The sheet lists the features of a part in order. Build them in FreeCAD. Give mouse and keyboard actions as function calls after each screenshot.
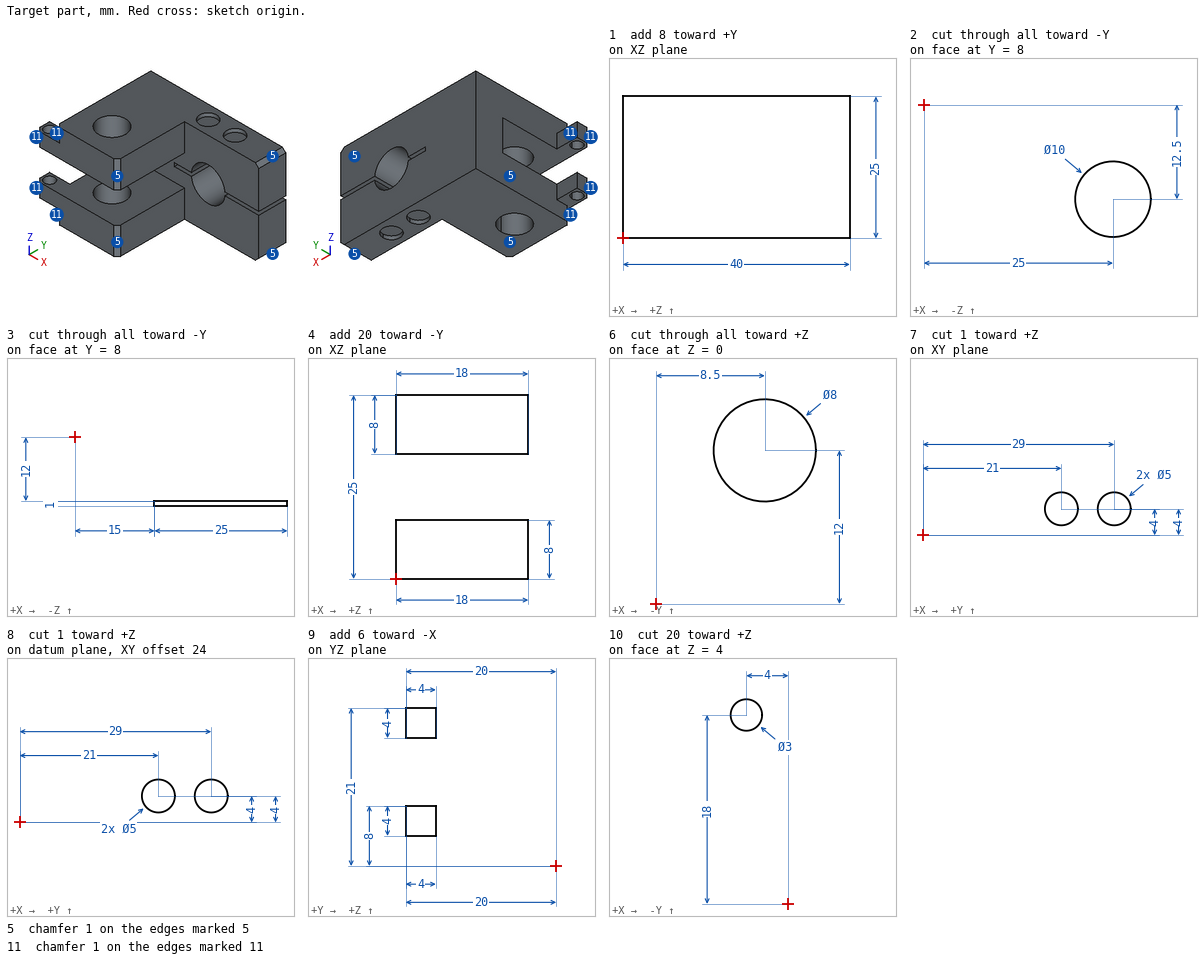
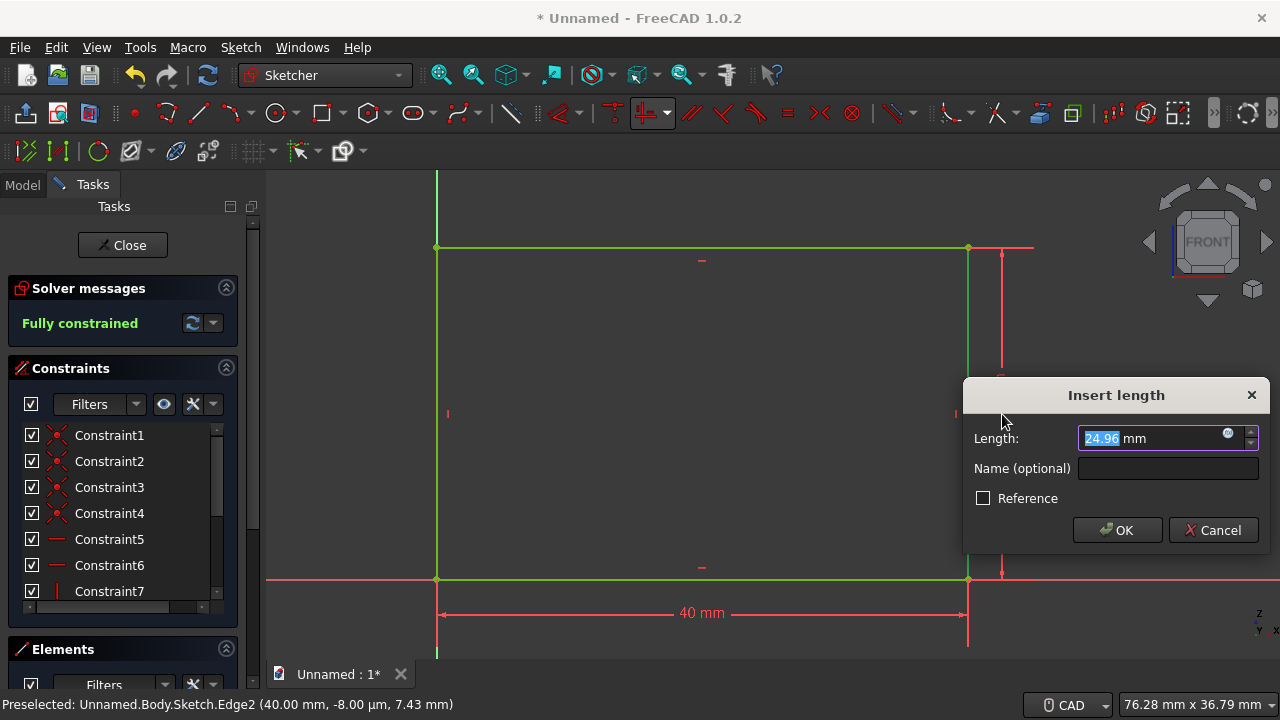
text(25)
key(Return)
key(Escape)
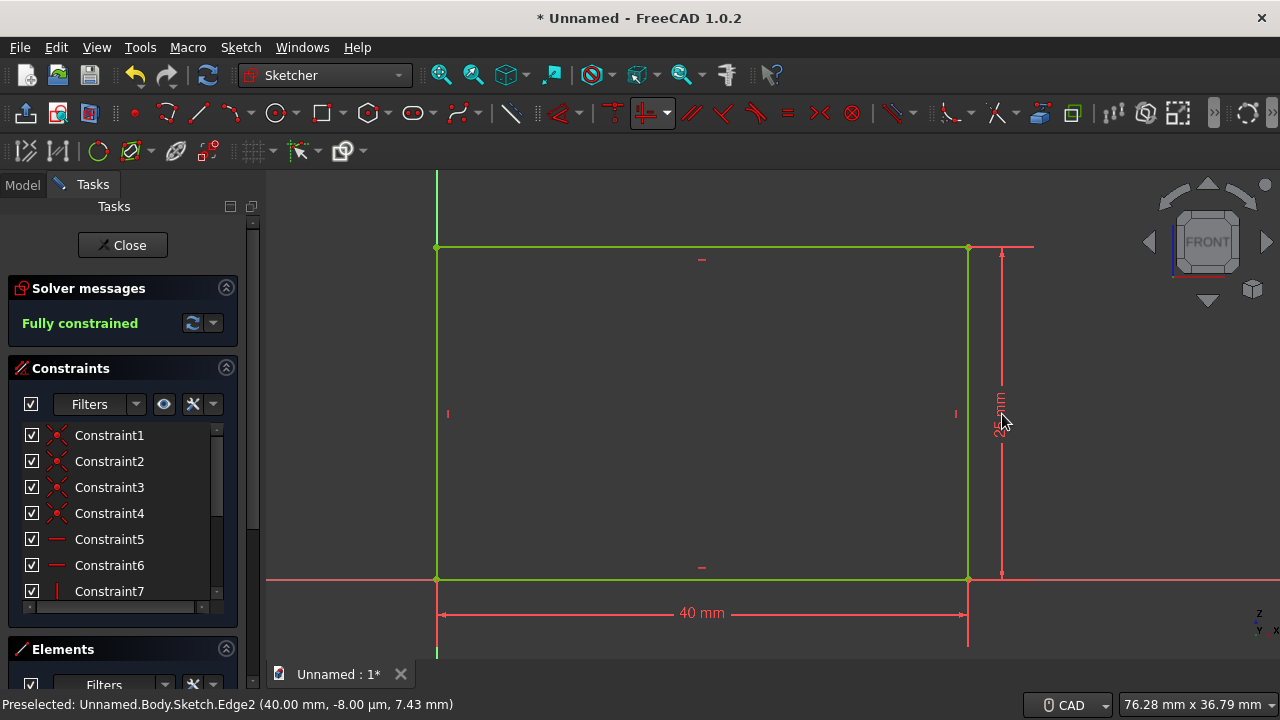
click(123, 245)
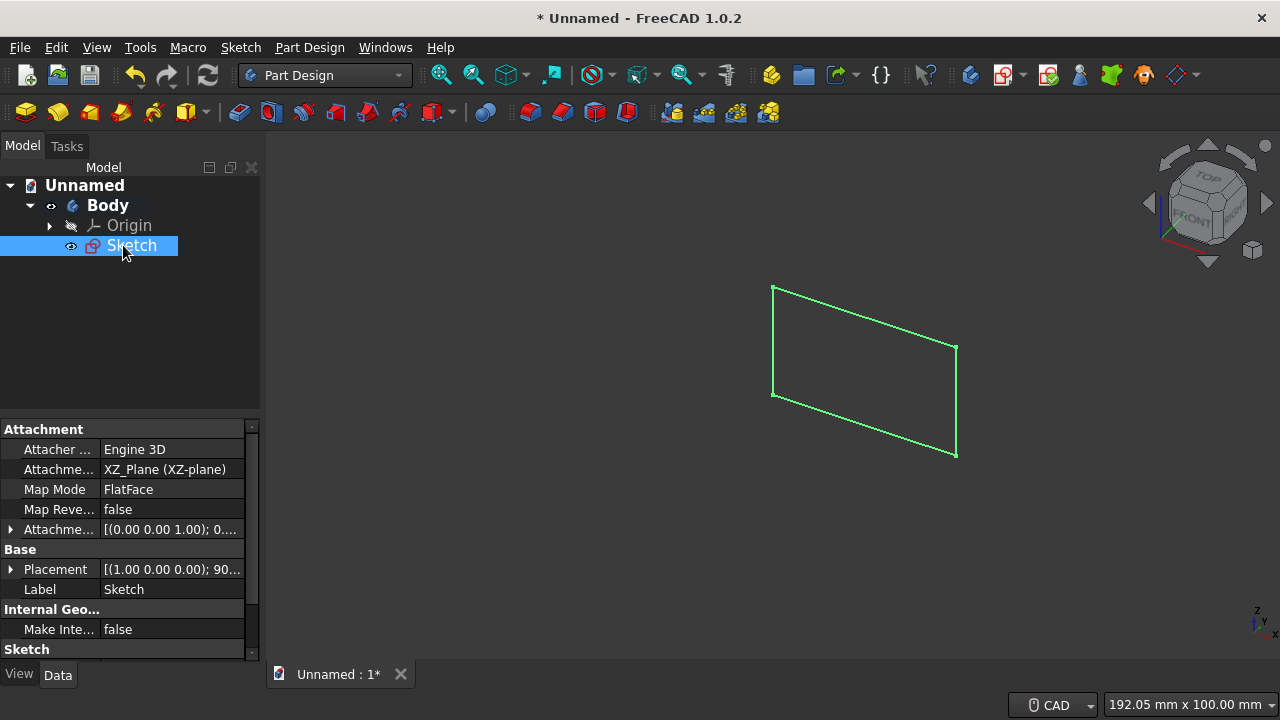
click(26, 112)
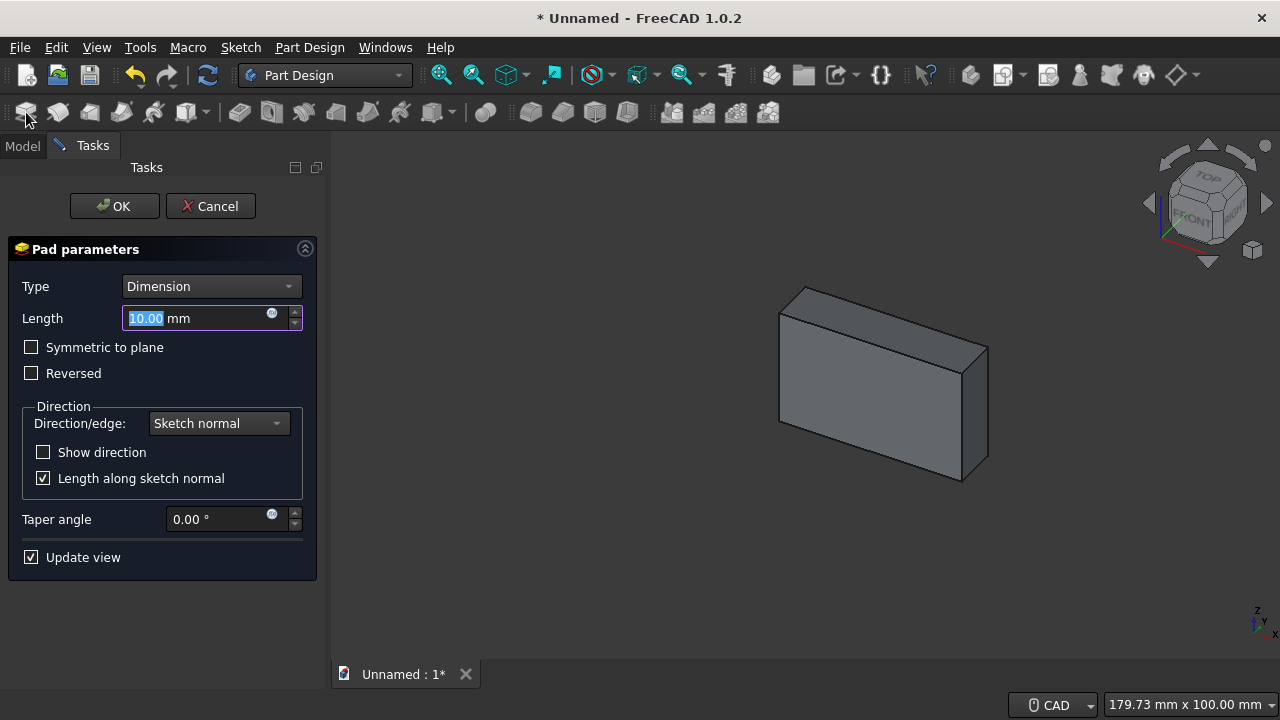
text(8)
key(Tab)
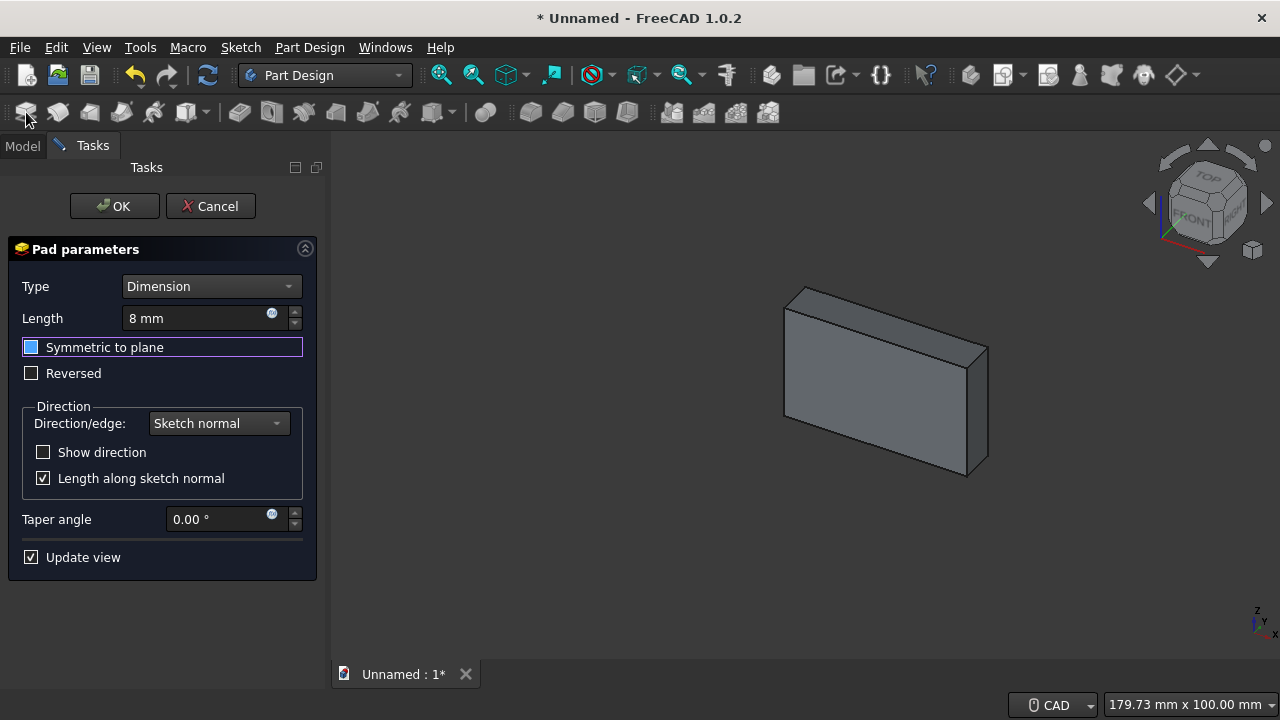
click(30, 373)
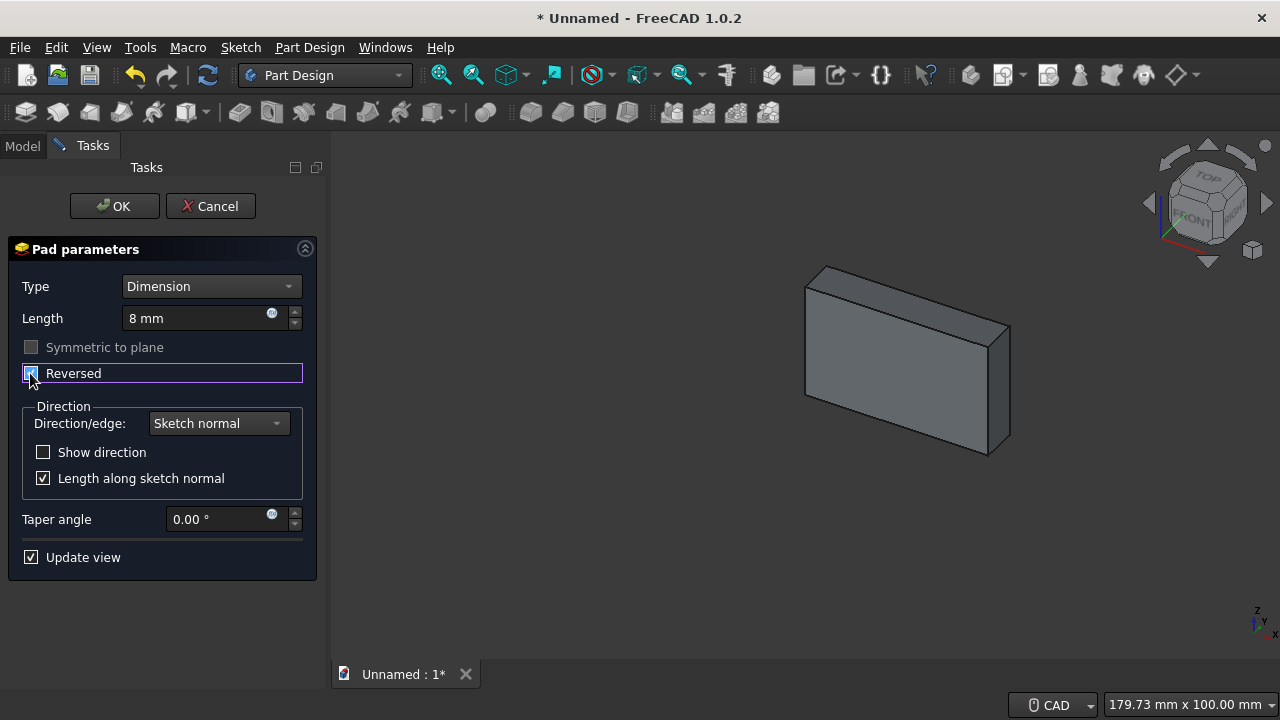
click(115, 206)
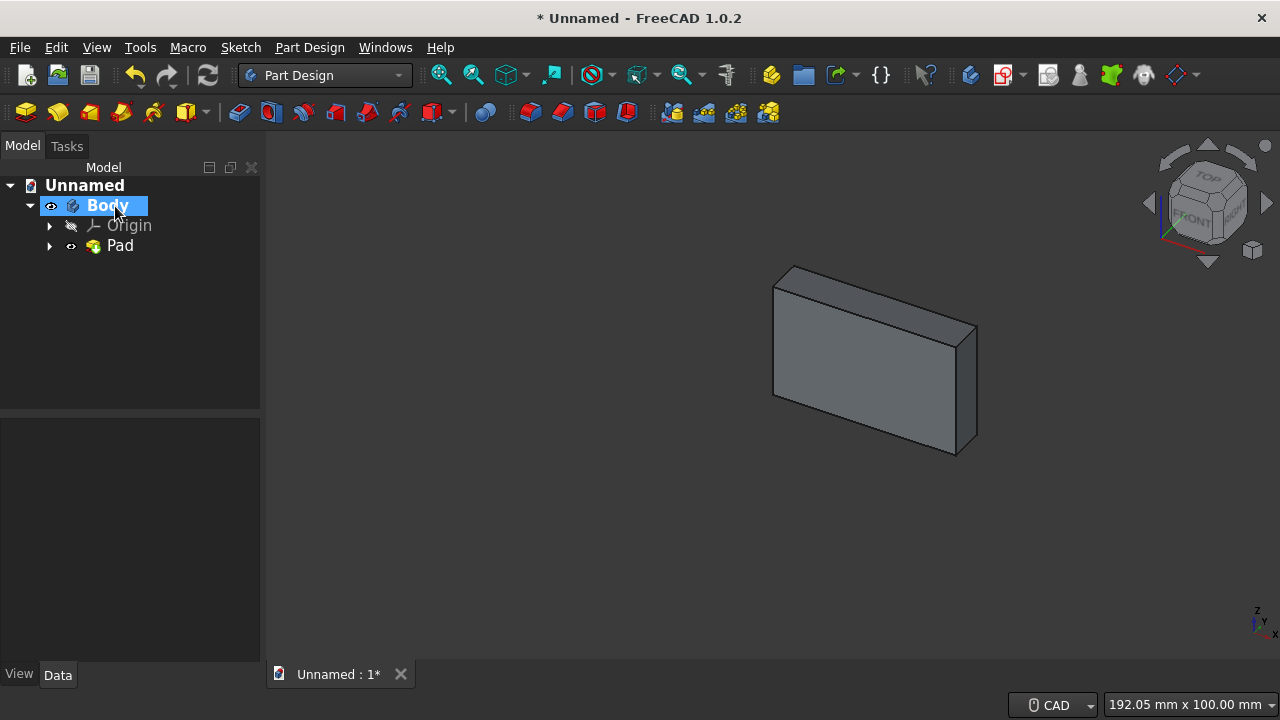
click(442, 76)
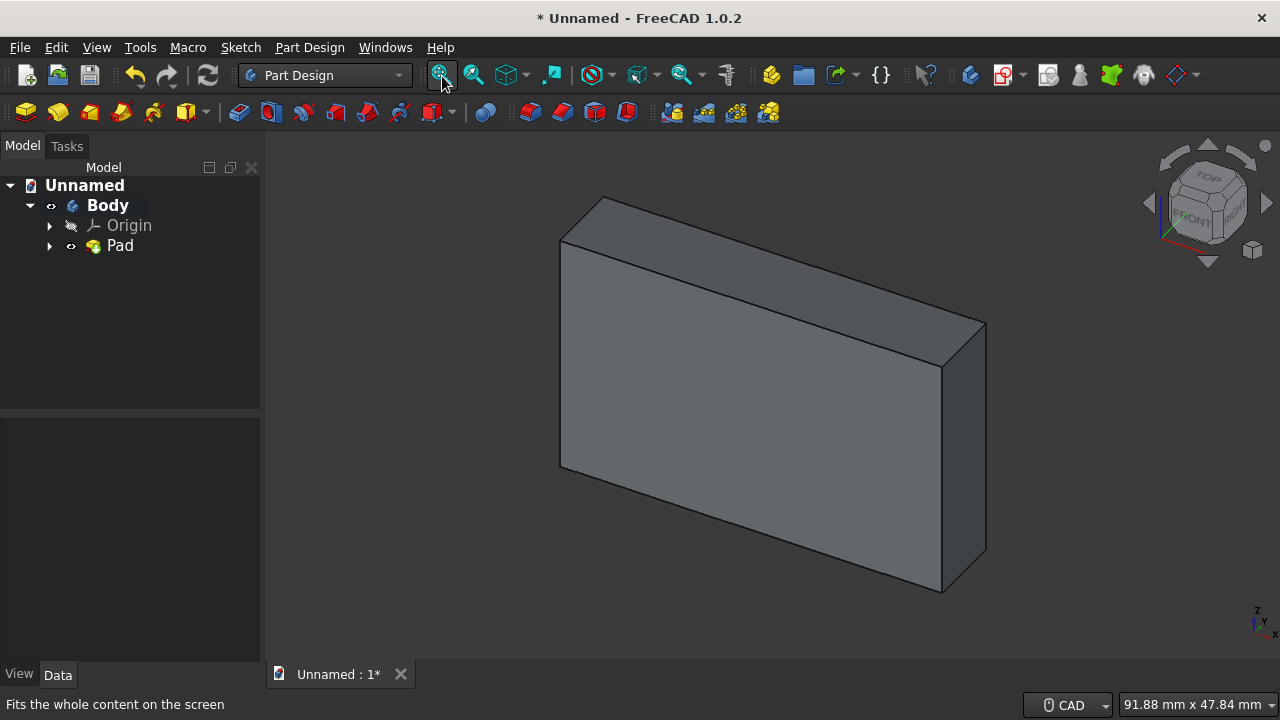
key(4)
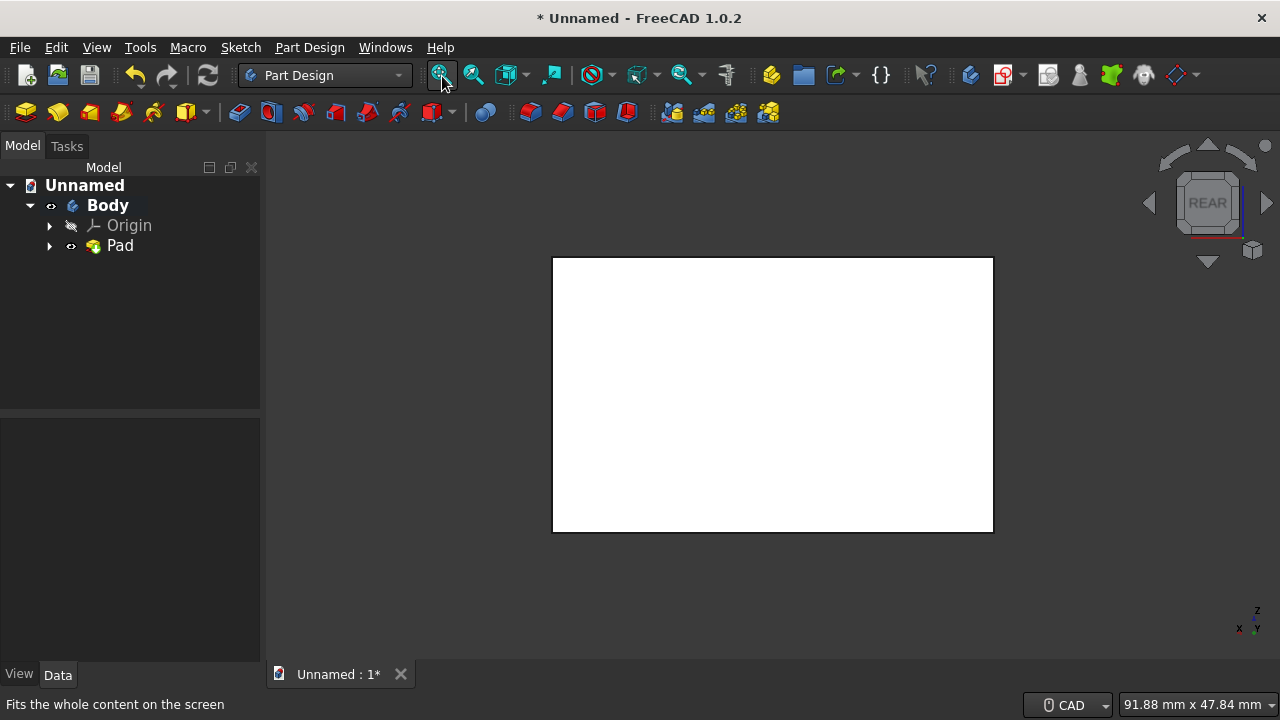
click(710, 394)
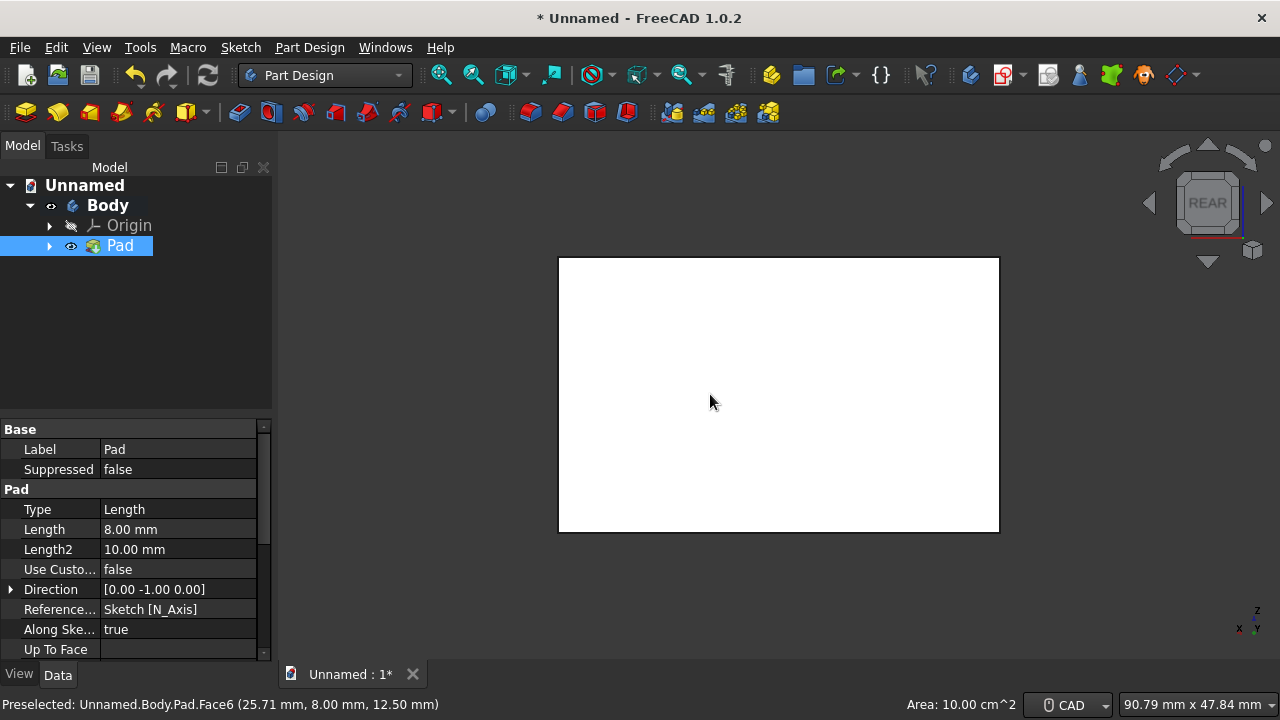
click(1004, 76)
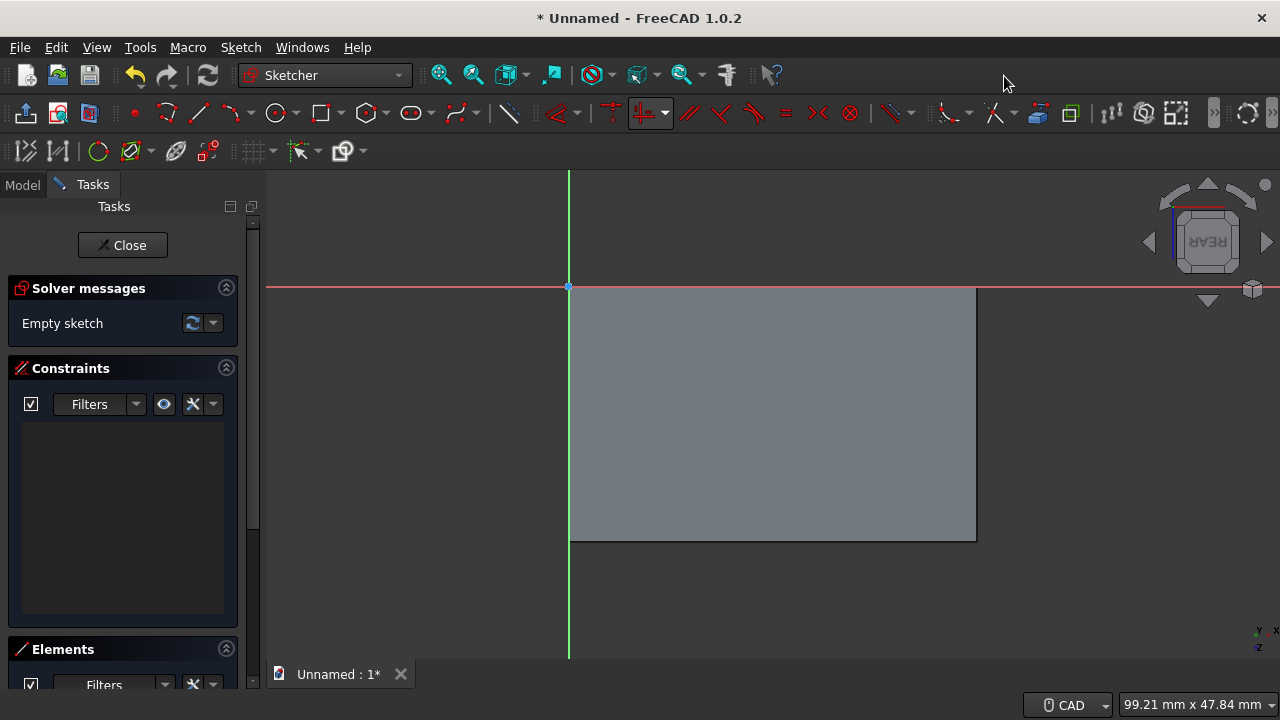
scroll(894, 414, up, 5)